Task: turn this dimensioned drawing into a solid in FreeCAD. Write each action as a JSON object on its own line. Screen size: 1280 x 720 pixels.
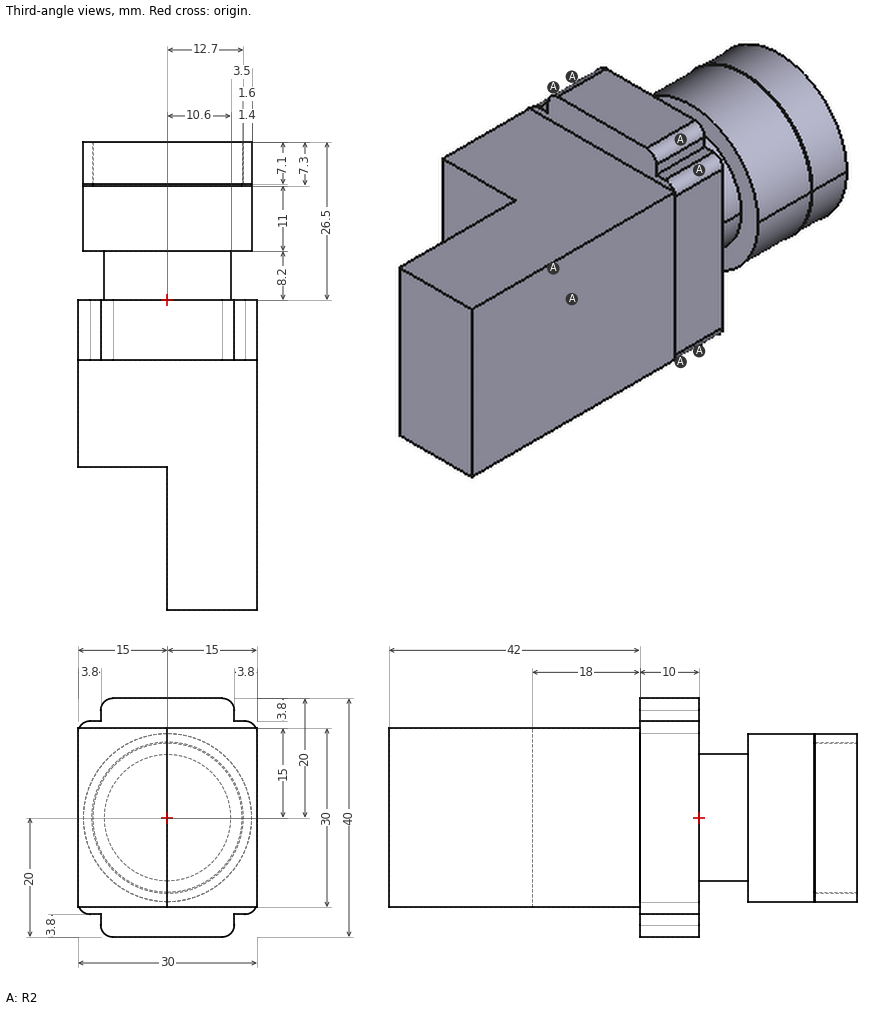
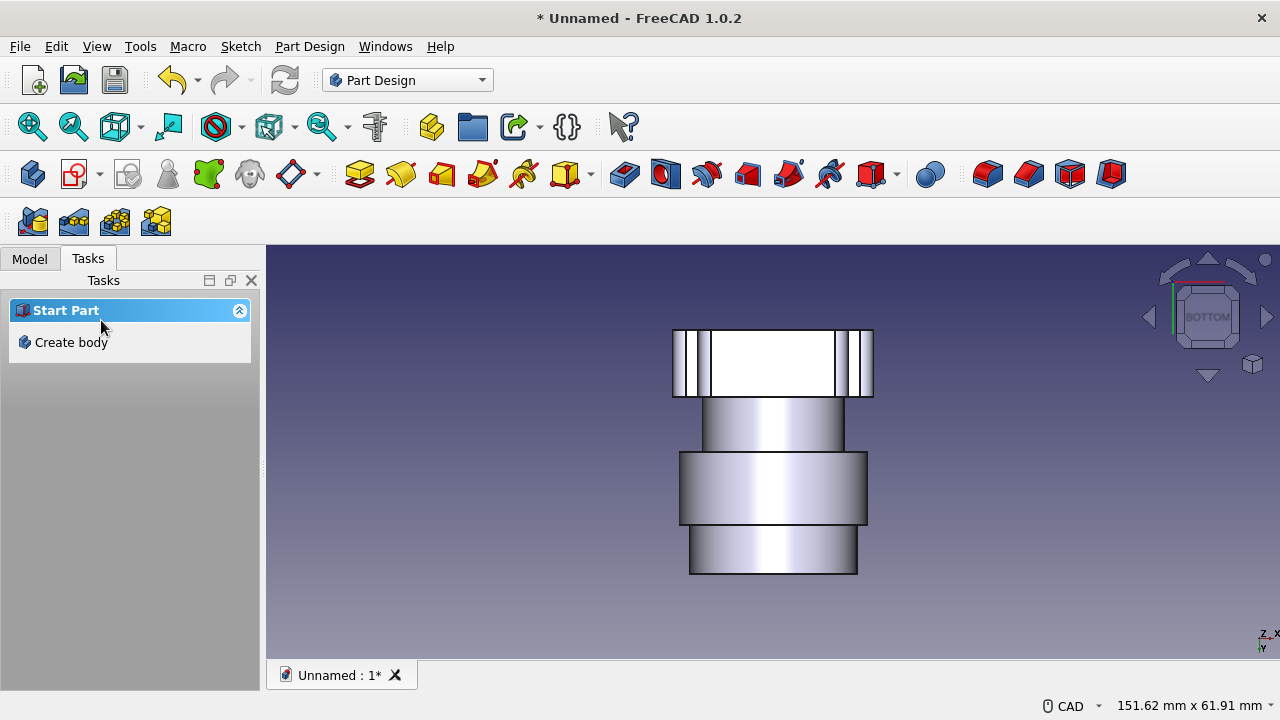
{"action": "left_click", "coordinate": [33, 174]}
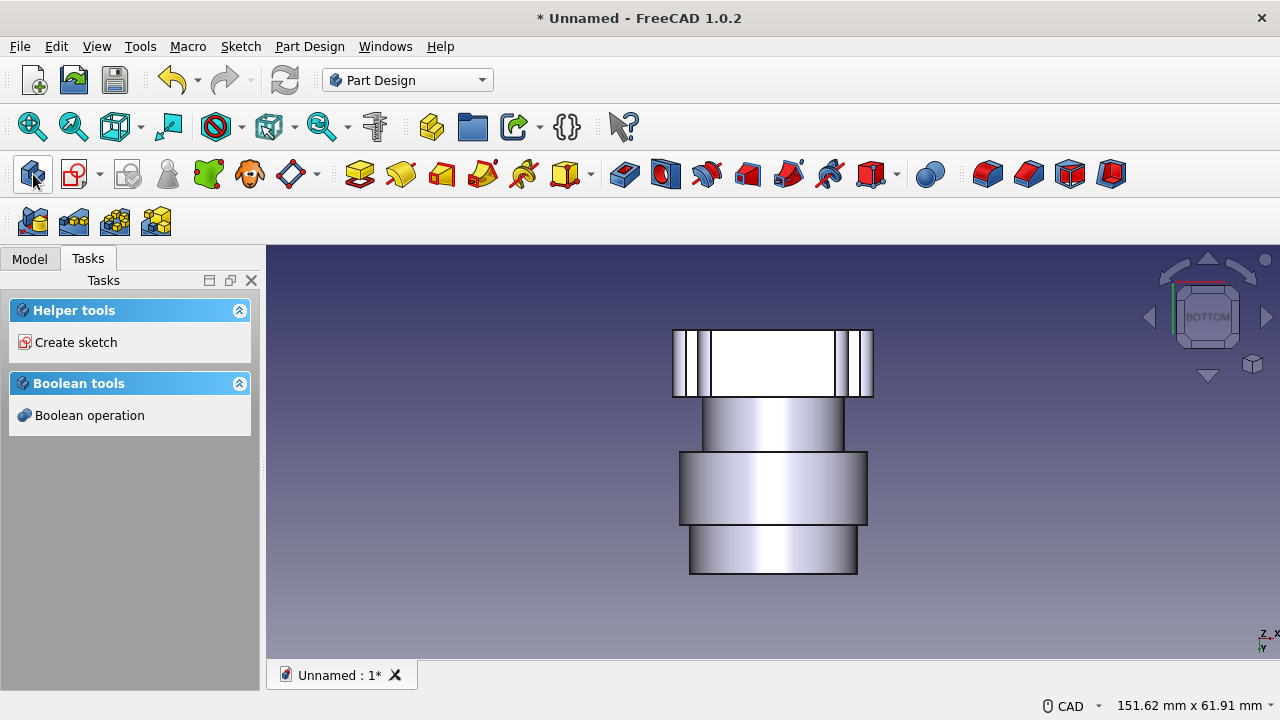
{"action": "left_click", "coordinate": [30, 258]}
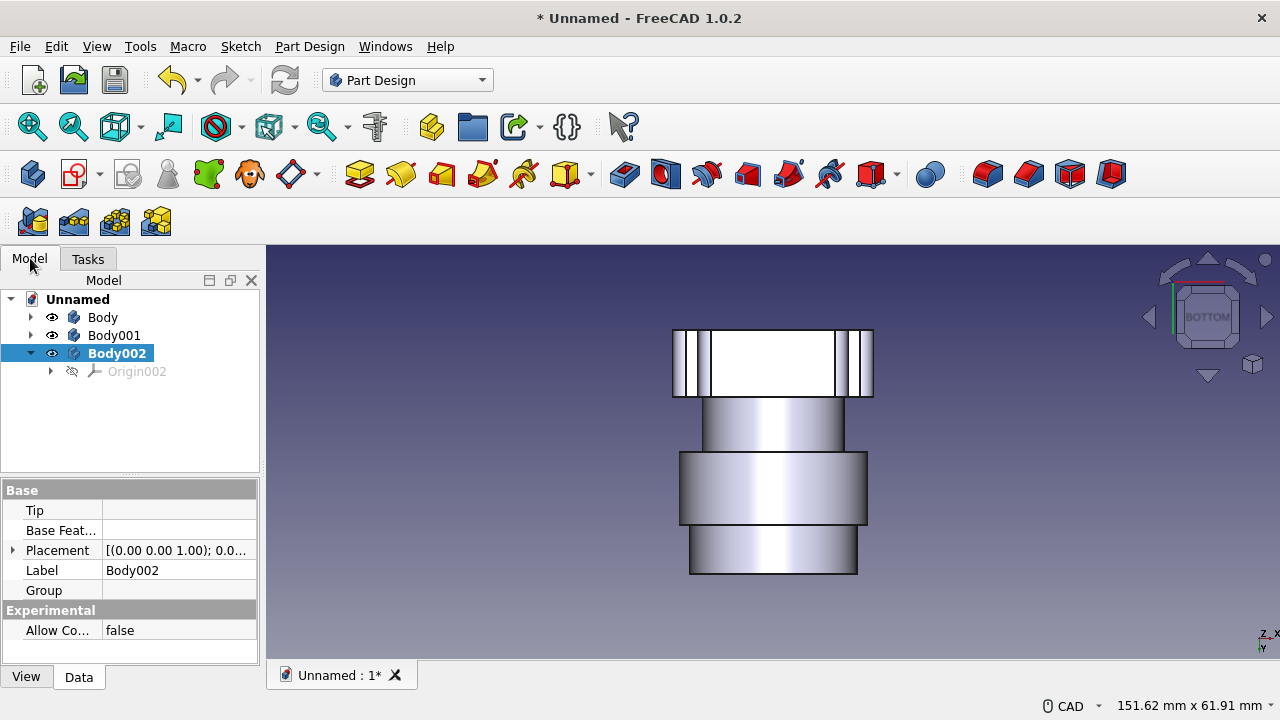
{"action": "left_click", "coordinate": [51, 371]}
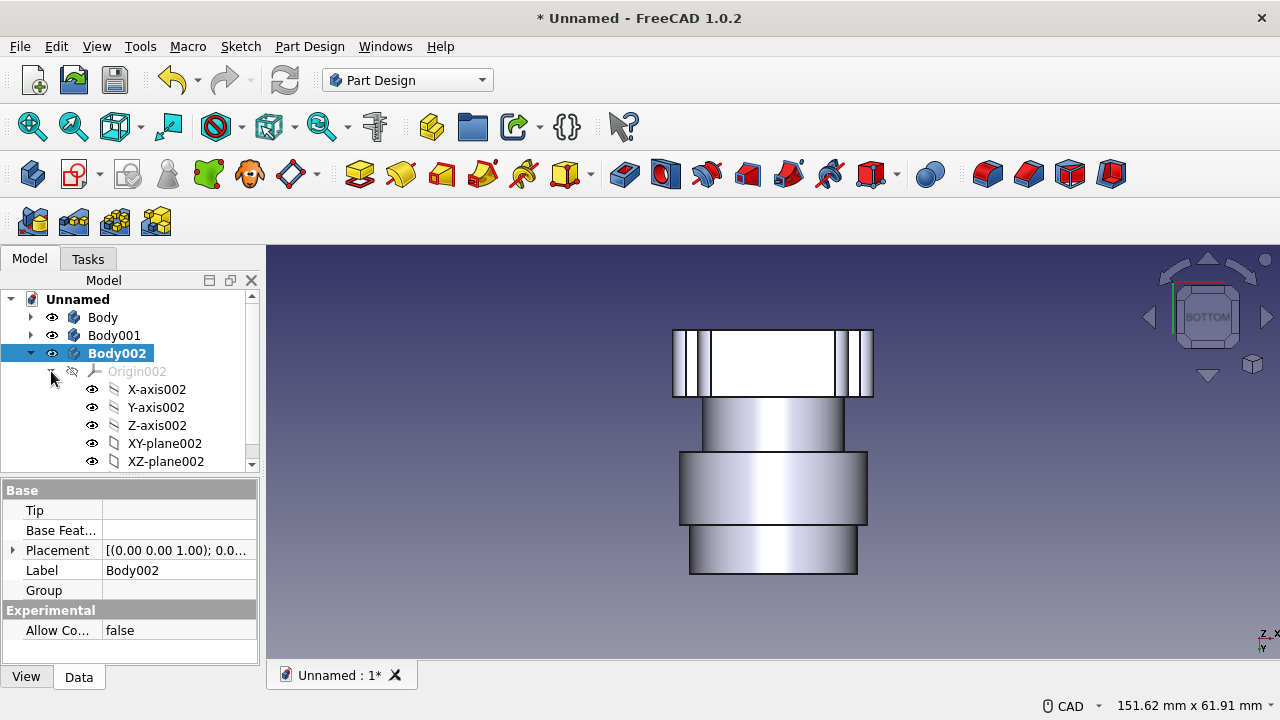
{"action": "left_click", "coordinate": [137, 461]}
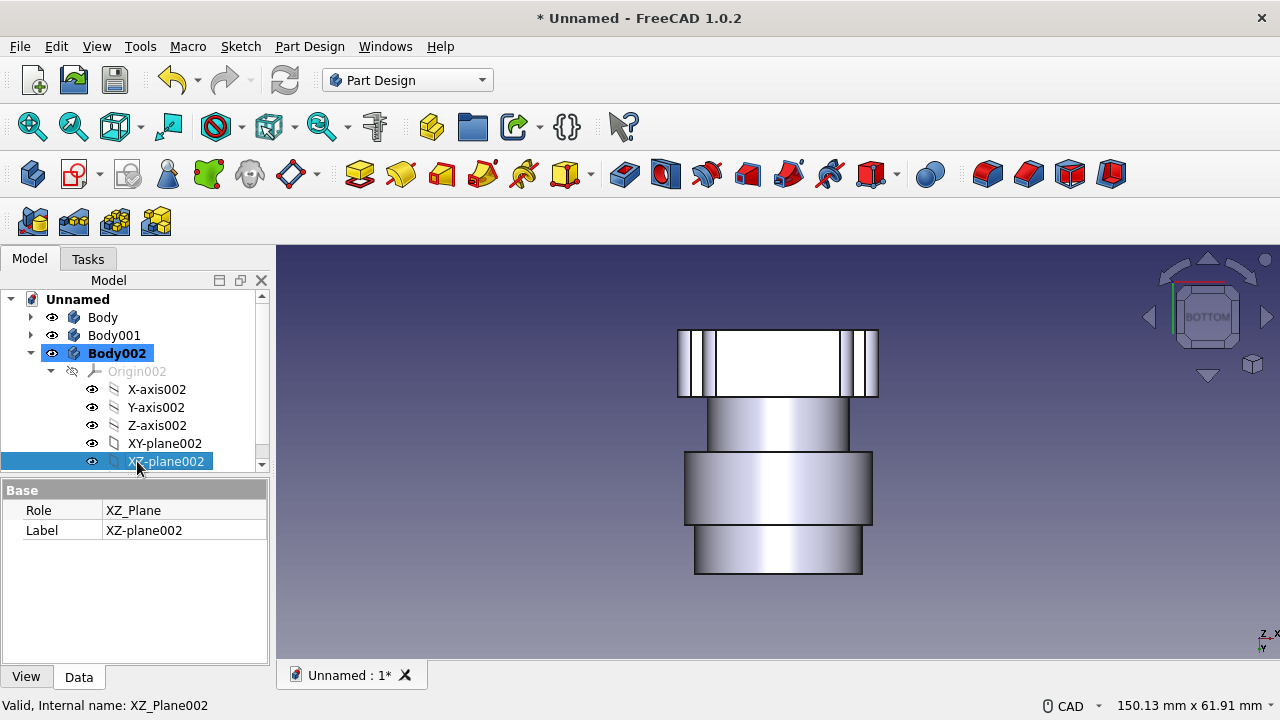
{"action": "left_click", "coordinate": [290, 174]}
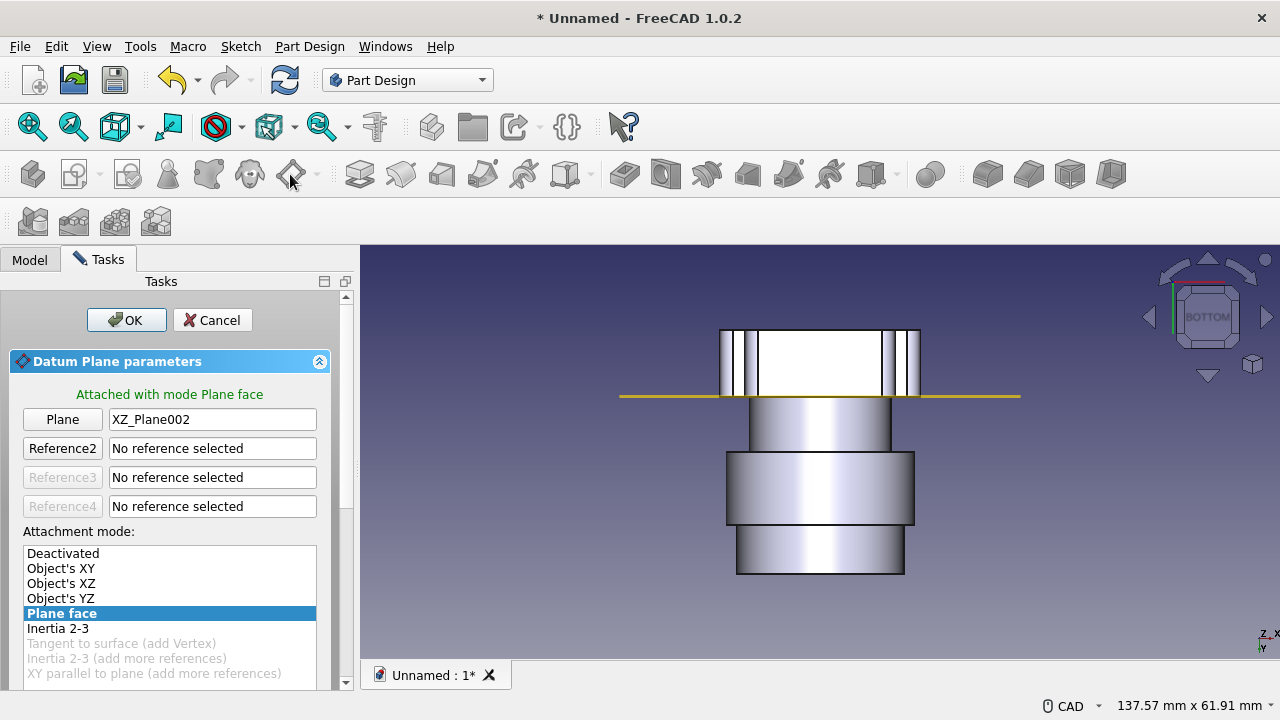
{"action": "scroll", "coordinate": [346, 490], "scroll_direction": "down", "scroll_amount": 4}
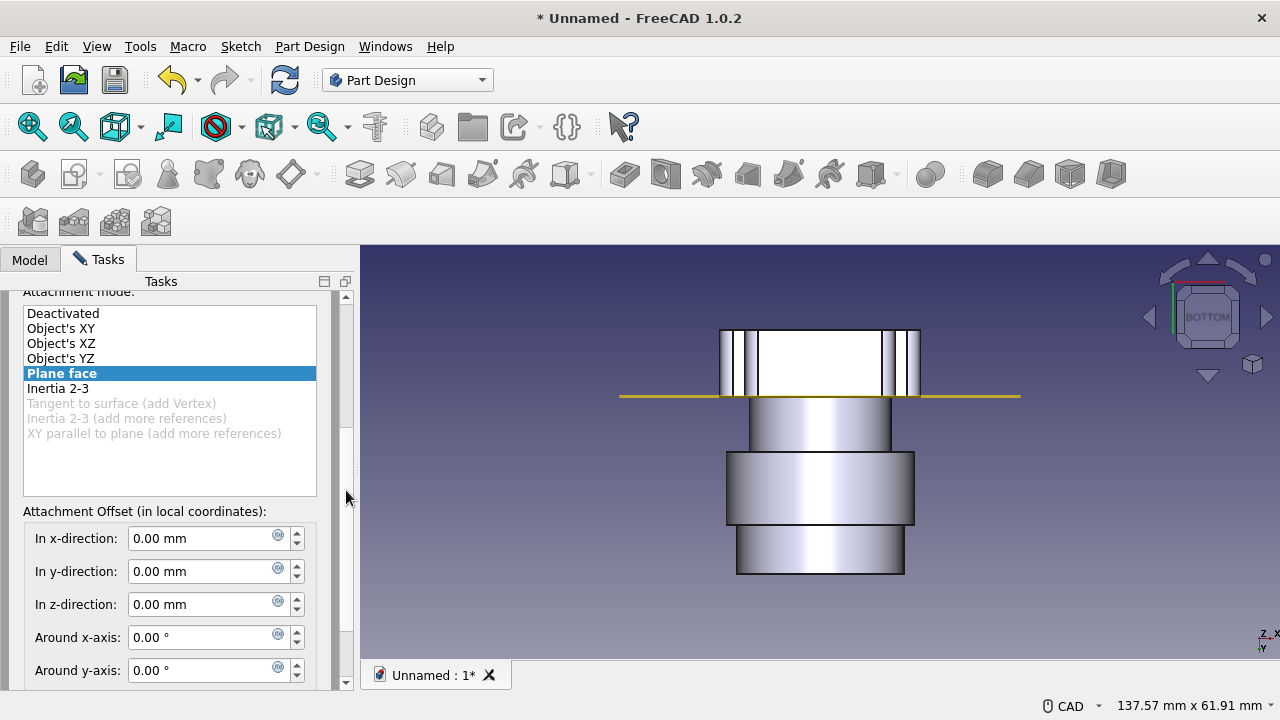
{"action": "triple_click", "coordinate": [210, 604]}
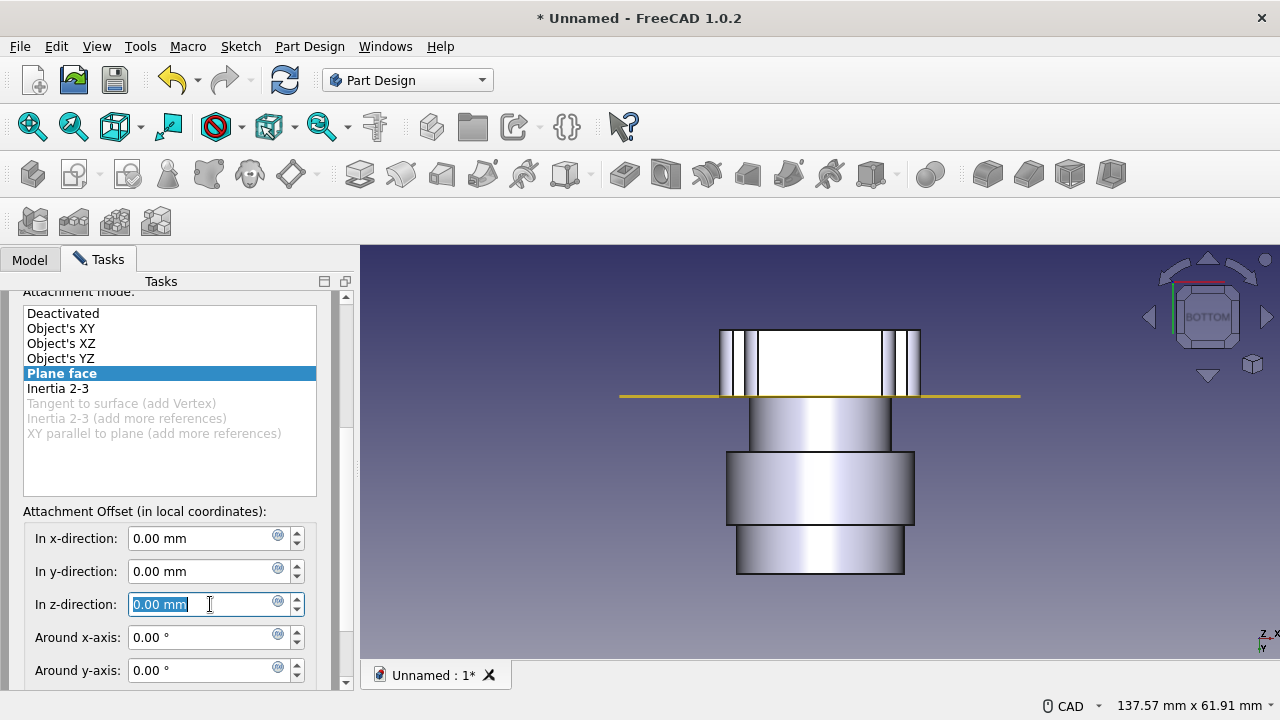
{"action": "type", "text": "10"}
{"action": "key", "text": "Tab"}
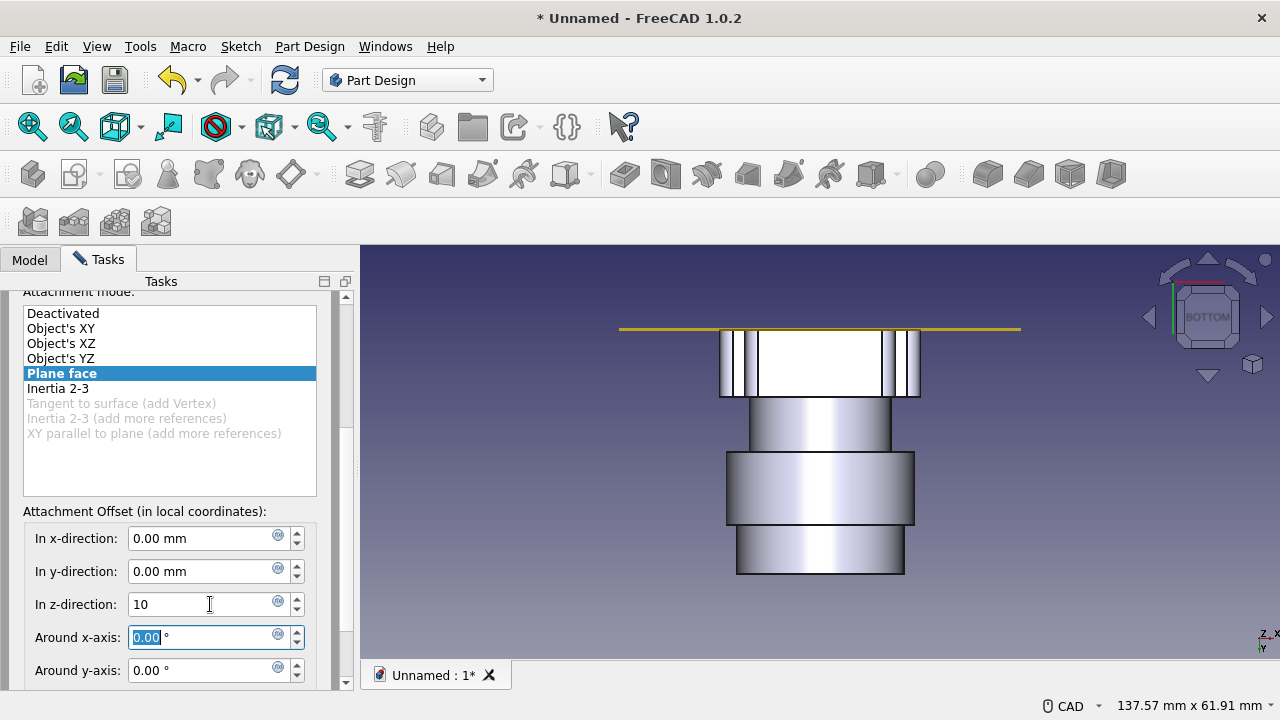
{"action": "scroll", "coordinate": [346, 490], "scroll_direction": "up", "scroll_amount": 5}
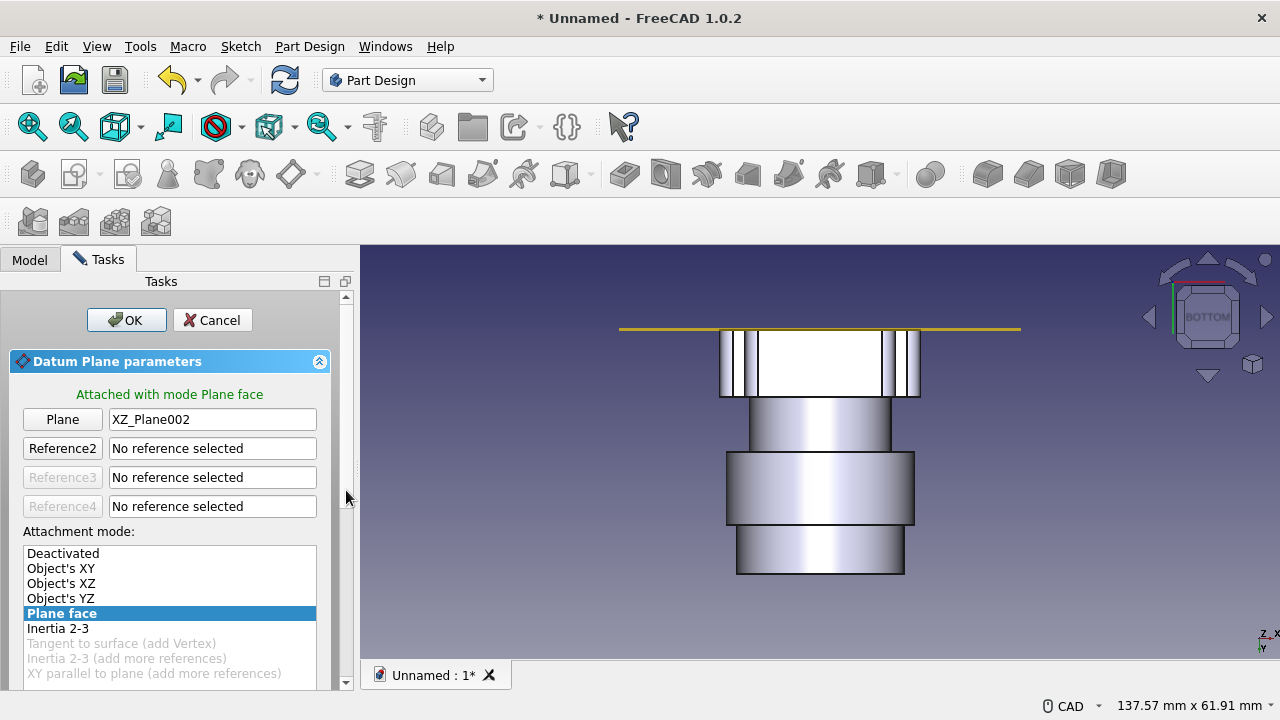
{"action": "left_click", "coordinate": [127, 320]}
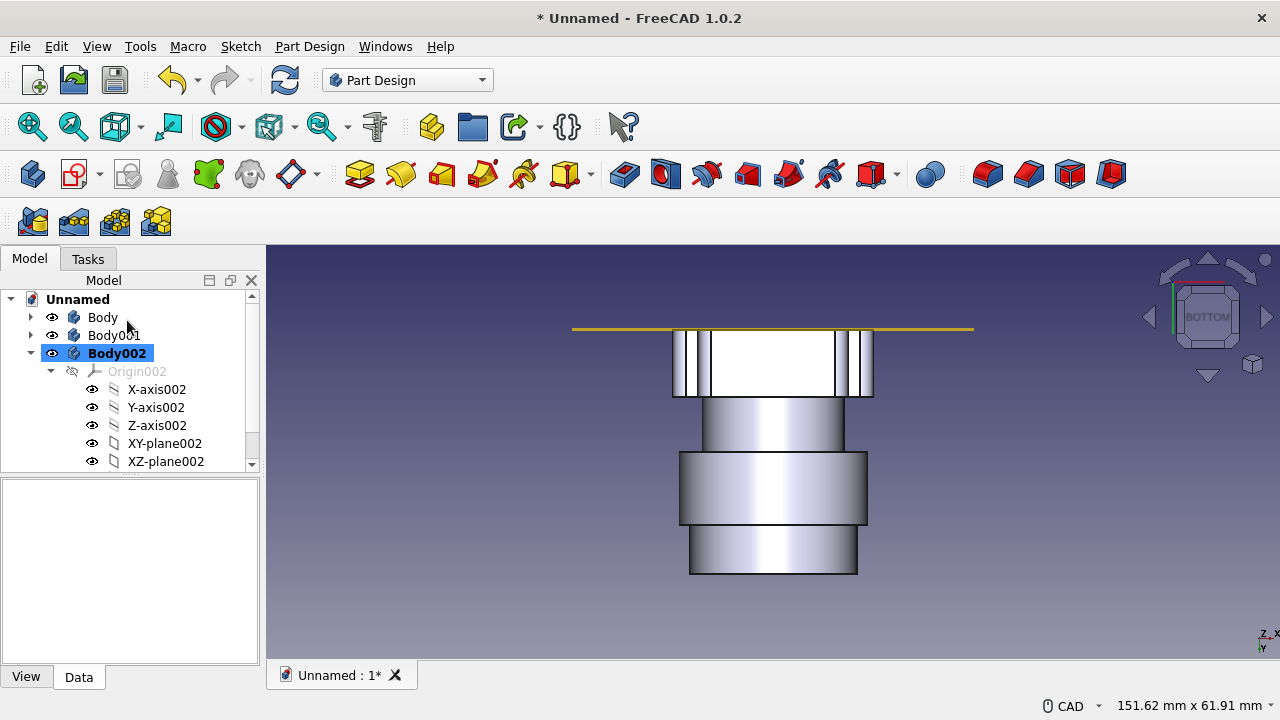
{"action": "scroll", "coordinate": [101, 385], "scroll_direction": "down", "scroll_amount": 3}